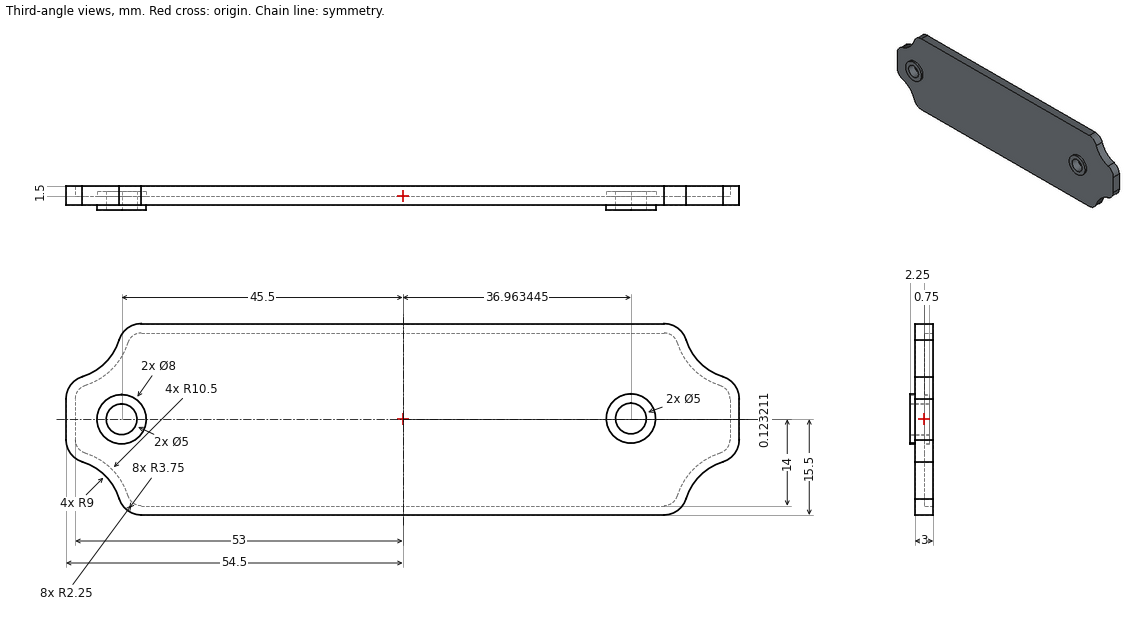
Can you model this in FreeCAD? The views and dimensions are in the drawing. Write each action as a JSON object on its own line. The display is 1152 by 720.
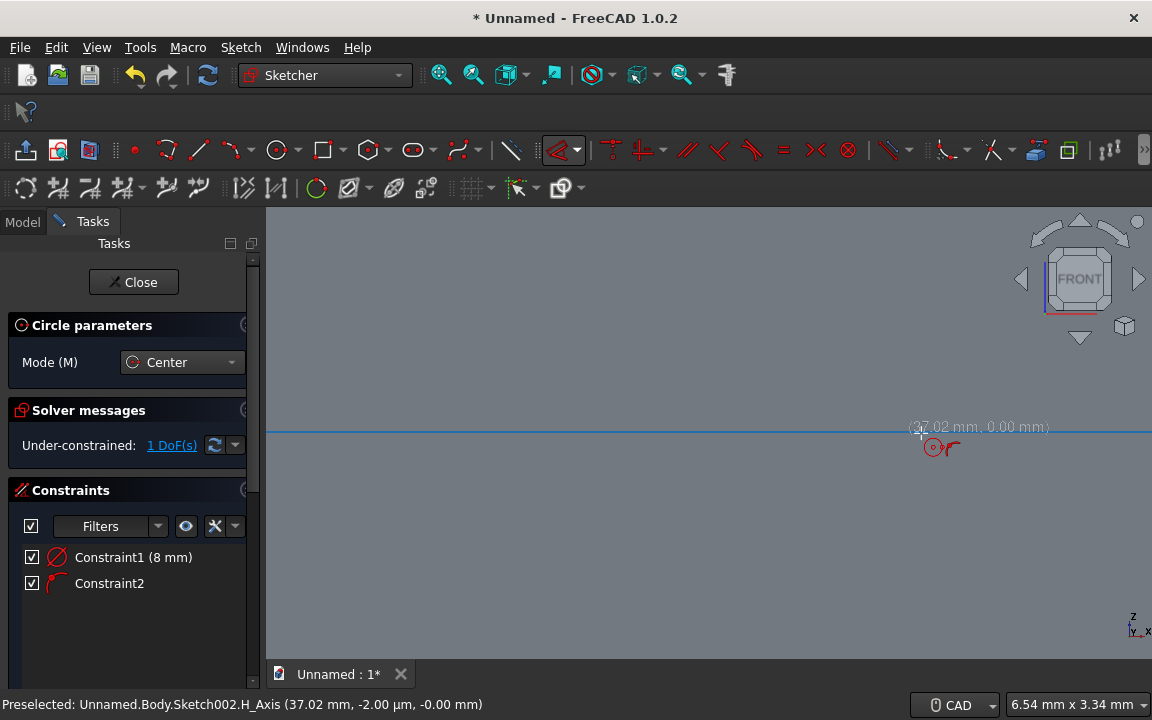
{"action": "left_click", "coordinate": [896, 415]}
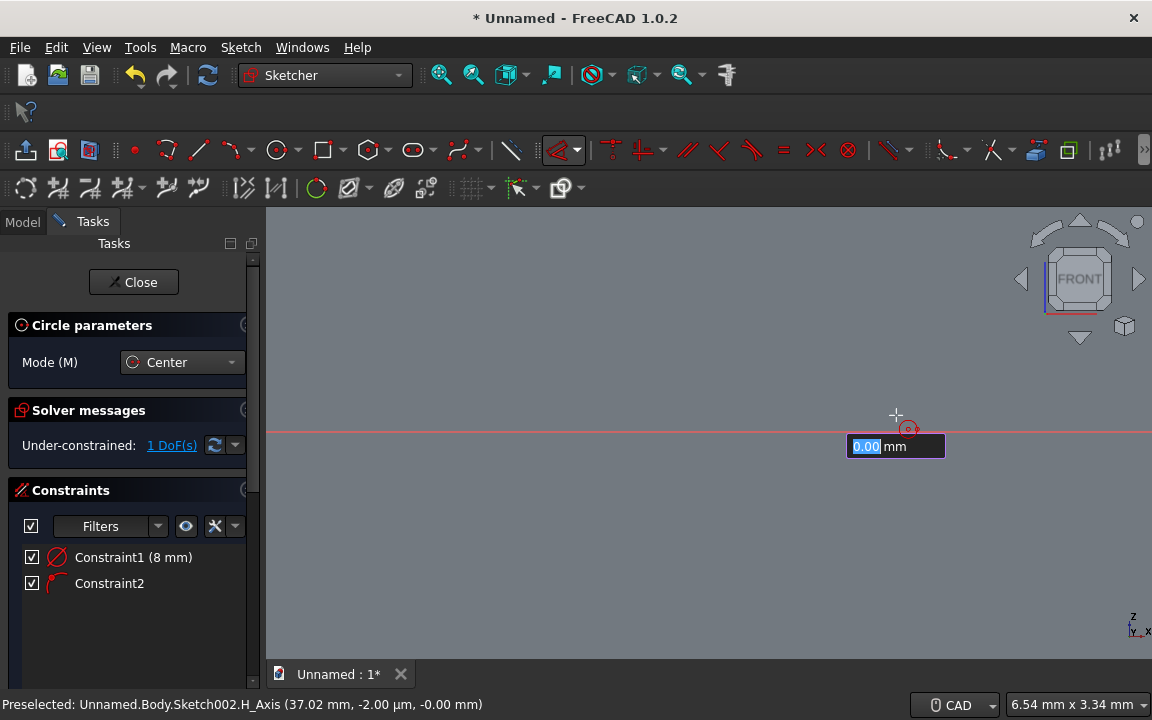
{"action": "scroll", "coordinate": [920, 433], "scroll_direction": "down", "scroll_amount": 15}
{"action": "mouse_move", "coordinate": [939, 414]}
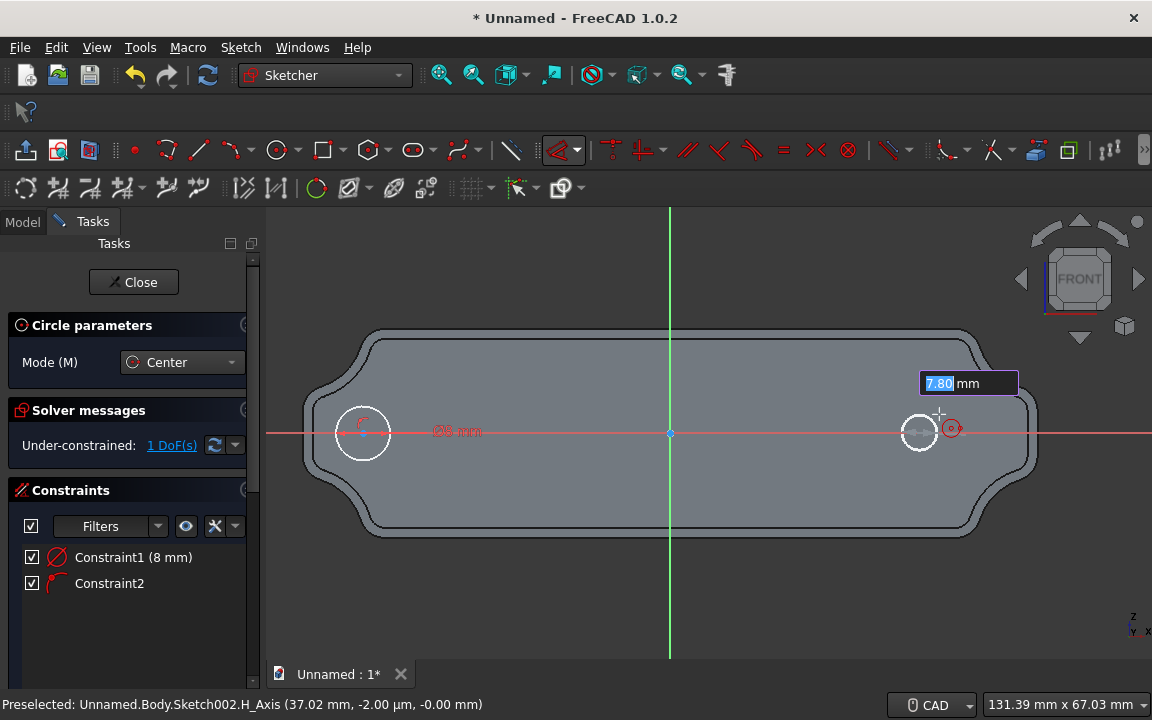
{"action": "type", "text": "8"}
{"action": "key", "text": "Return"}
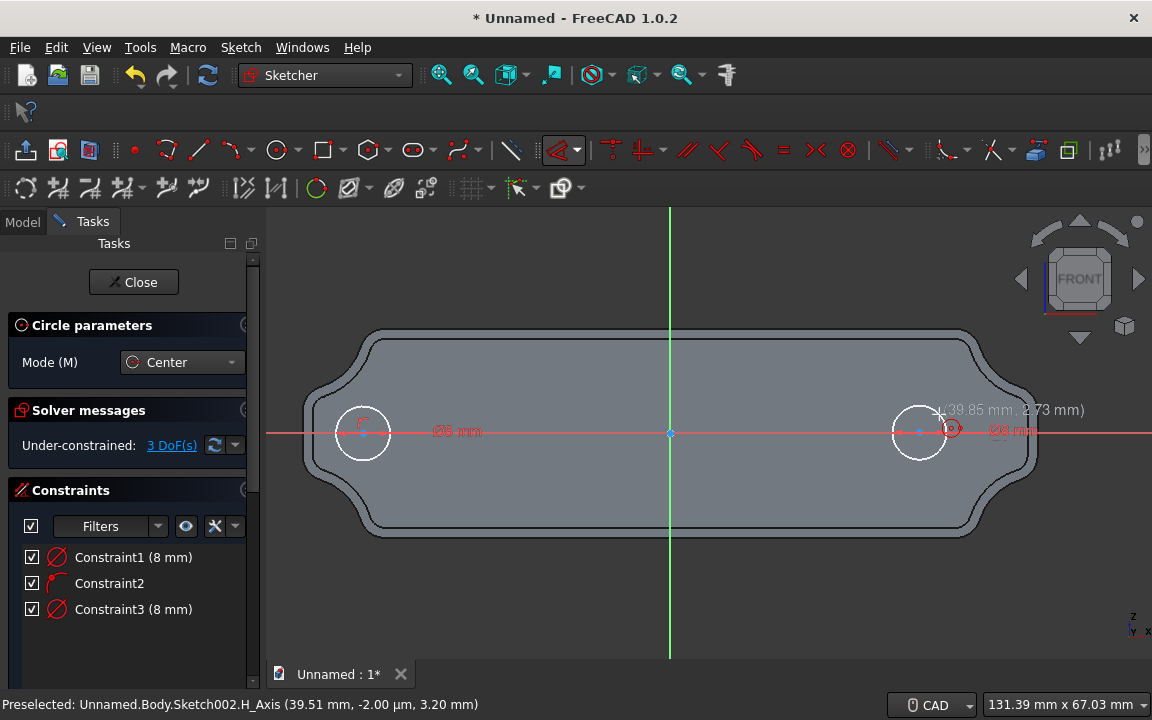
{"action": "scroll", "coordinate": [363, 433], "scroll_direction": "up", "scroll_amount": 2}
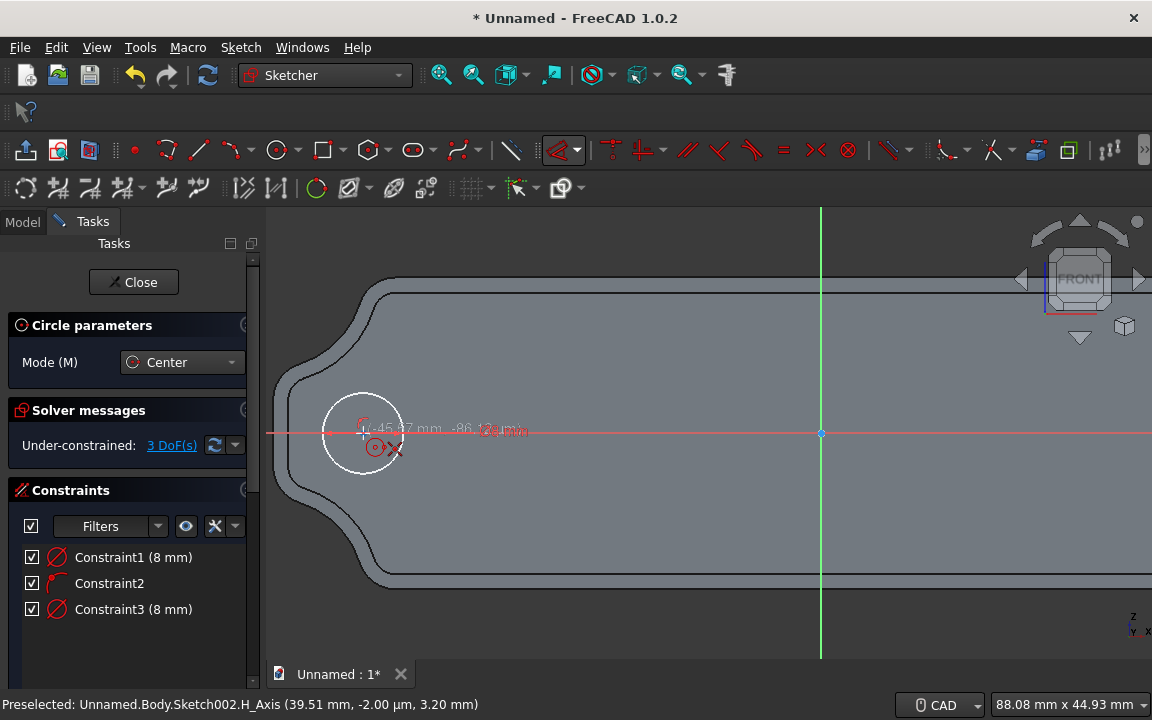
{"action": "left_click", "coordinate": [363, 433]}
{"action": "mouse_move", "coordinate": [381, 416]}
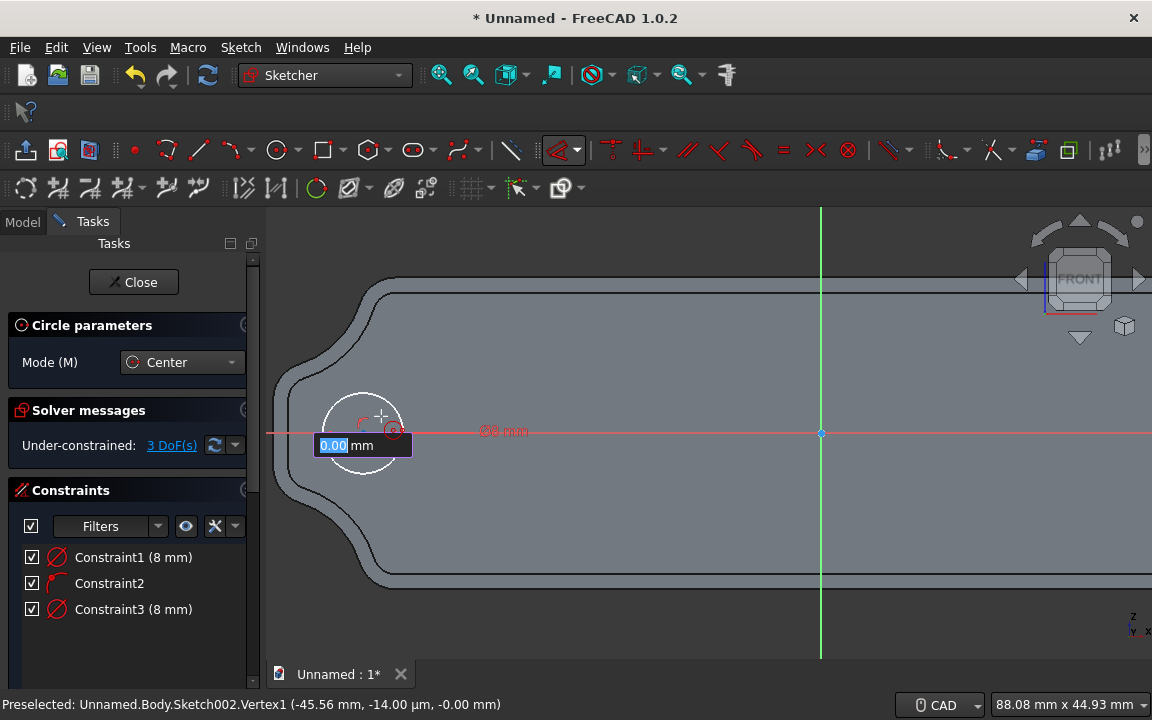
{"action": "type", "text": "5"}
{"action": "key", "text": "Return"}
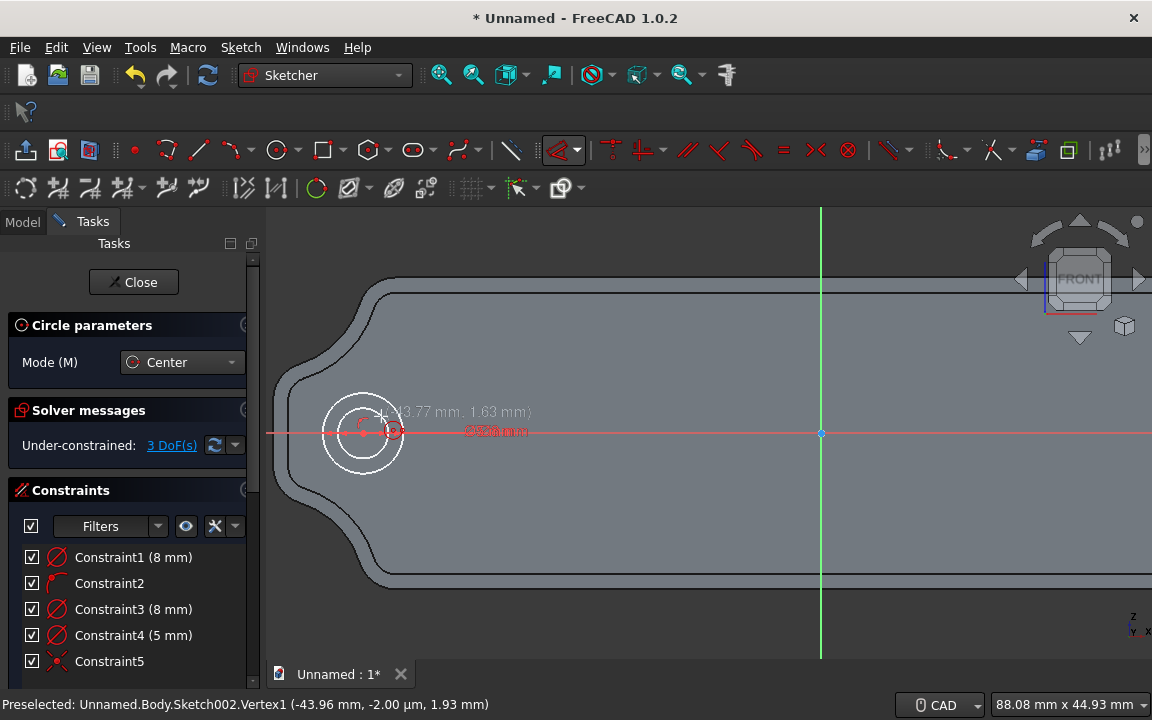
{"action": "scroll", "coordinate": [473, 433], "scroll_direction": "down", "scroll_amount": 3}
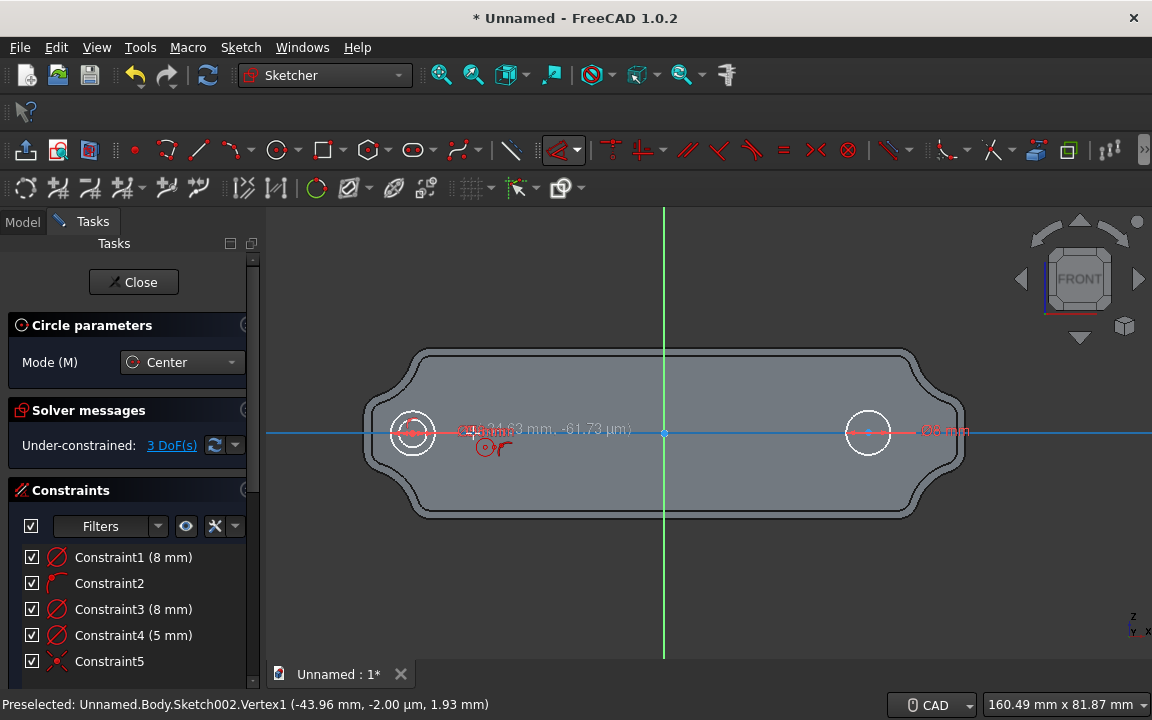
{"action": "scroll", "coordinate": [868, 433], "scroll_direction": "up", "scroll_amount": 16}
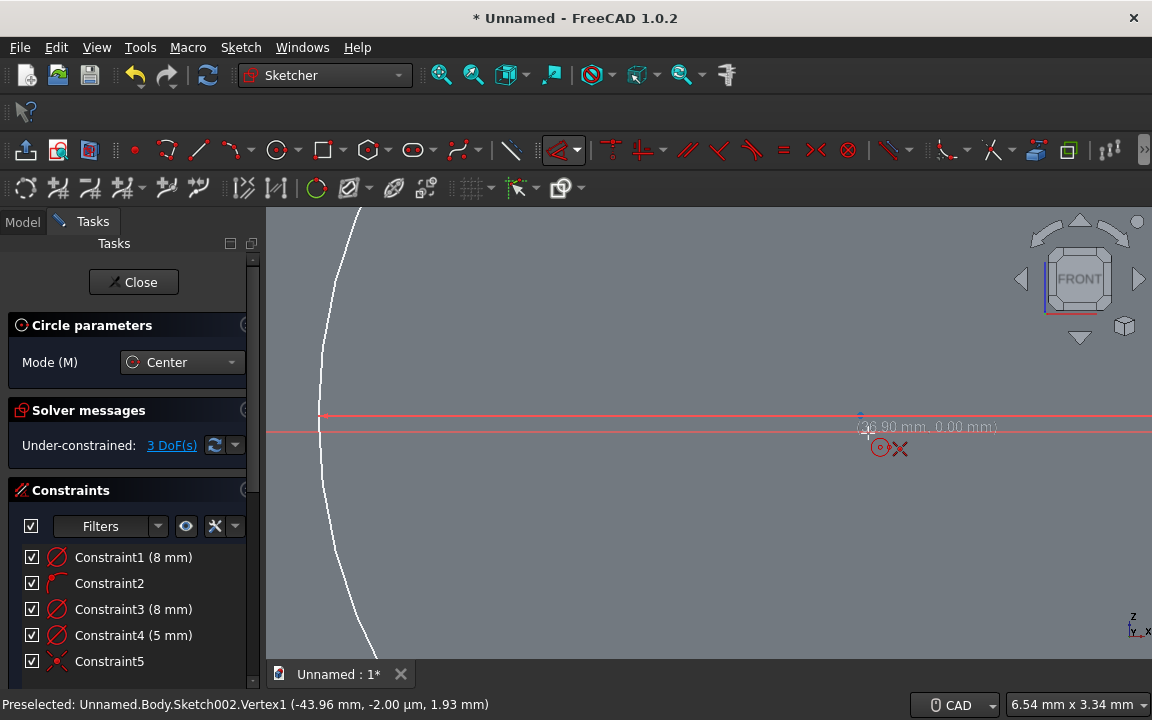
{"action": "left_click", "coordinate": [860, 416]}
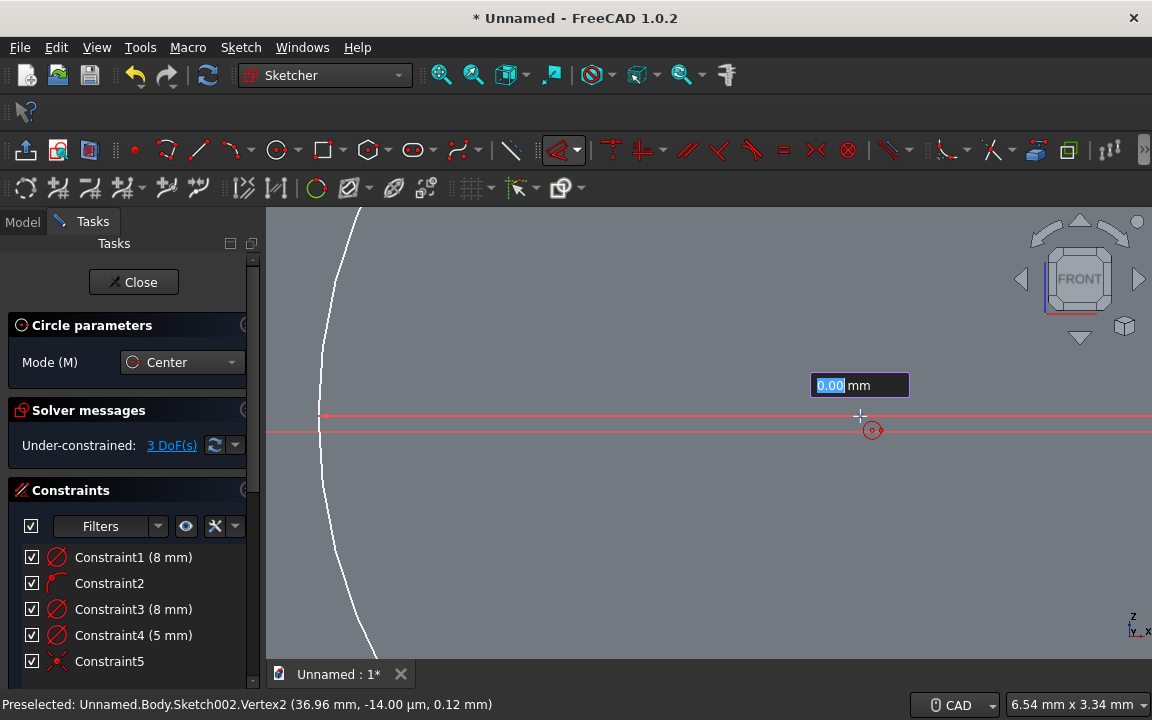
{"action": "scroll", "coordinate": [922, 433], "scroll_direction": "down", "scroll_amount": 15}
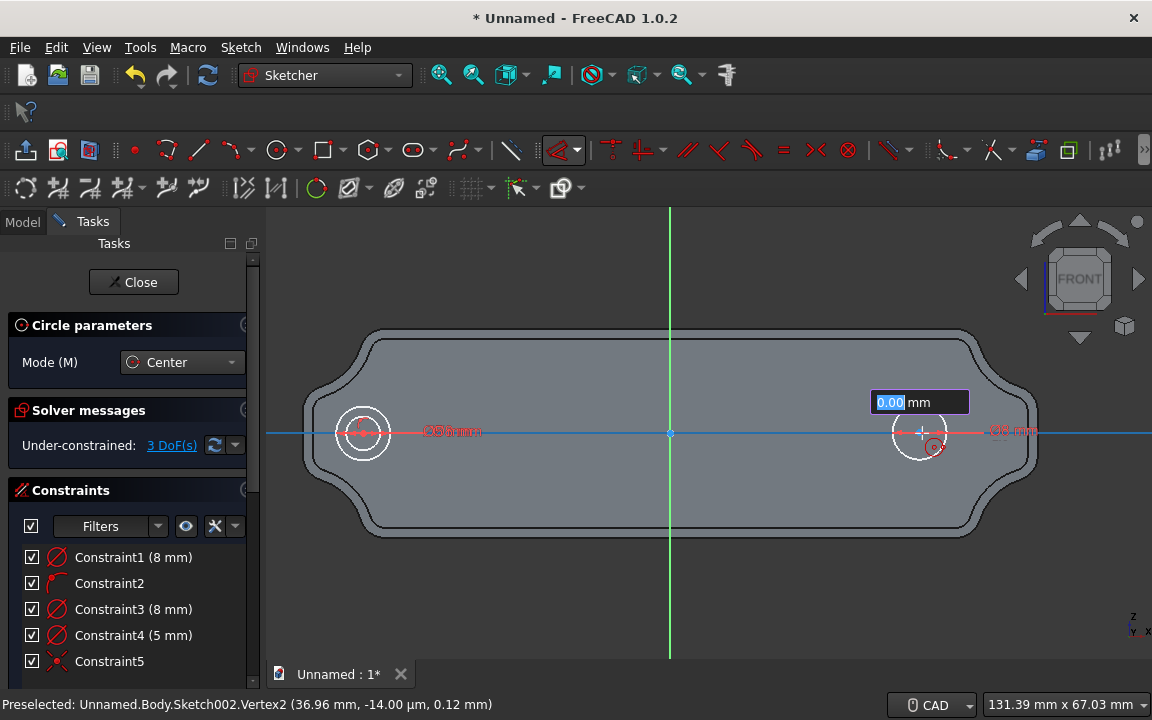
{"action": "scroll", "coordinate": [932, 421], "scroll_direction": "up", "scroll_amount": 3}
{"action": "mouse_move", "coordinate": [931, 420]}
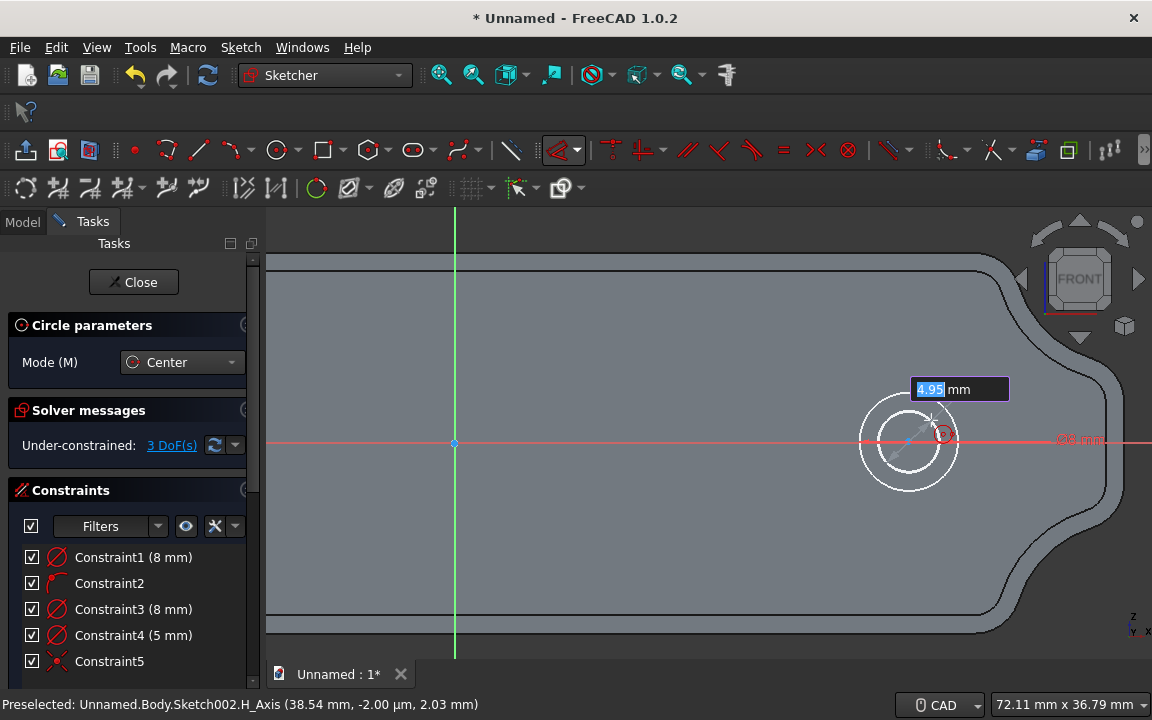
{"action": "type", "text": "5"}
{"action": "key", "text": "Return"}
{"action": "key", "text": "Escape"}